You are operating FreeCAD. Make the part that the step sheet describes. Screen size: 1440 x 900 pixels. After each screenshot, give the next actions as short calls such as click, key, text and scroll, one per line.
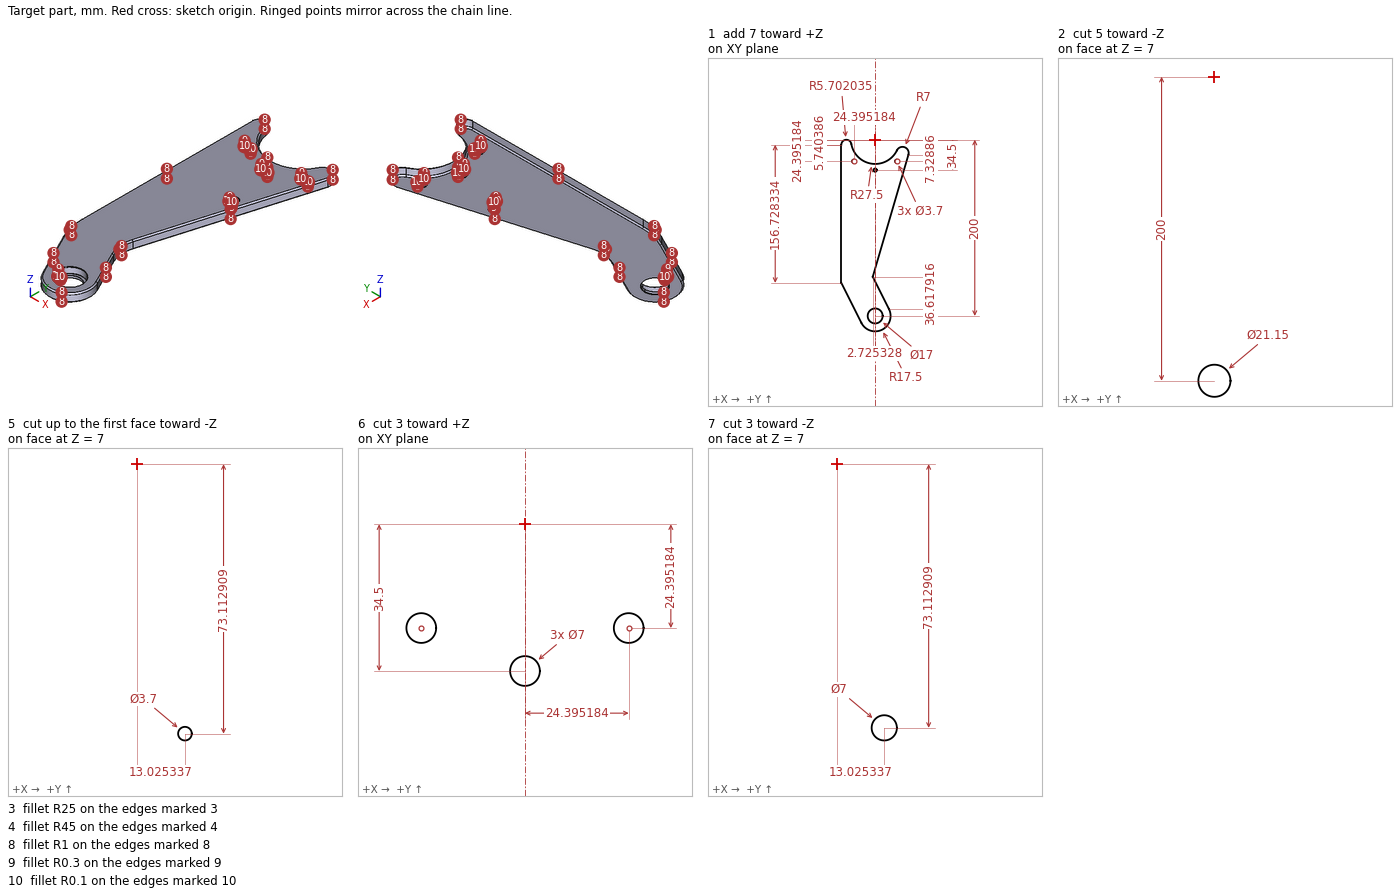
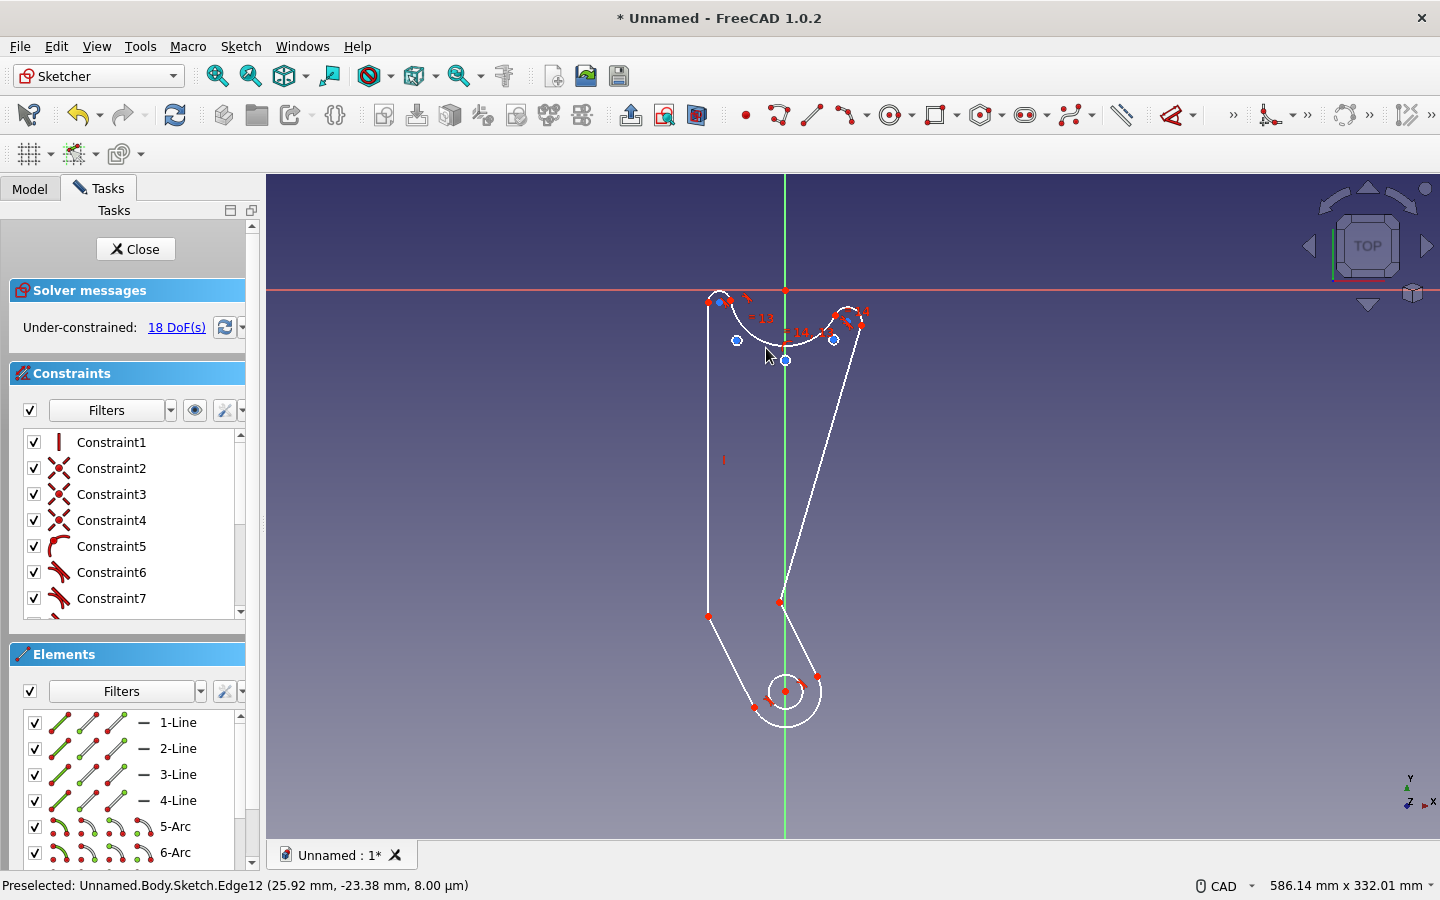
click(786, 692)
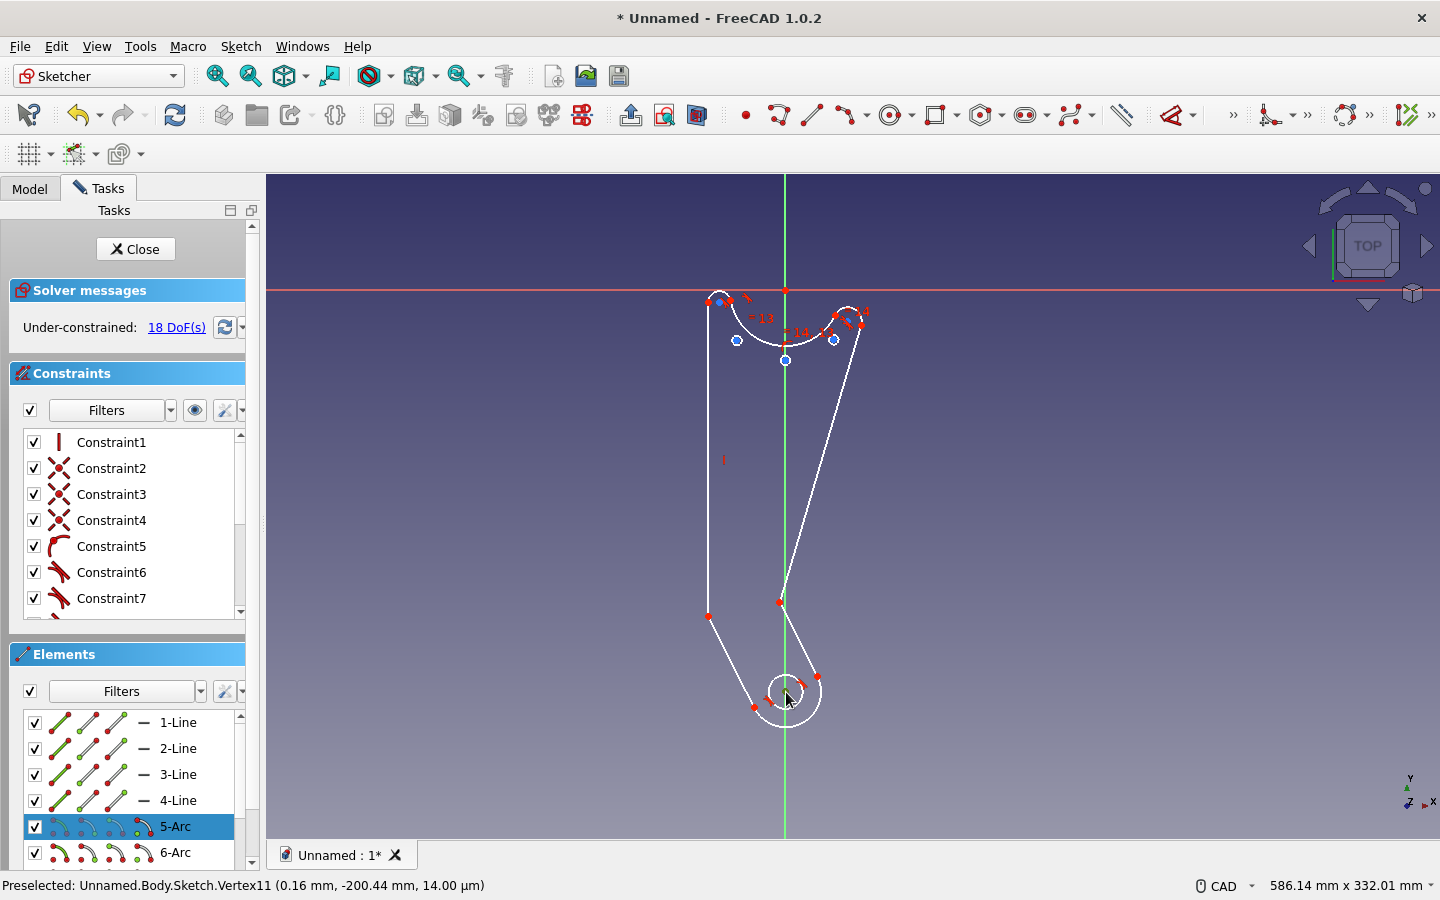
click(785, 768)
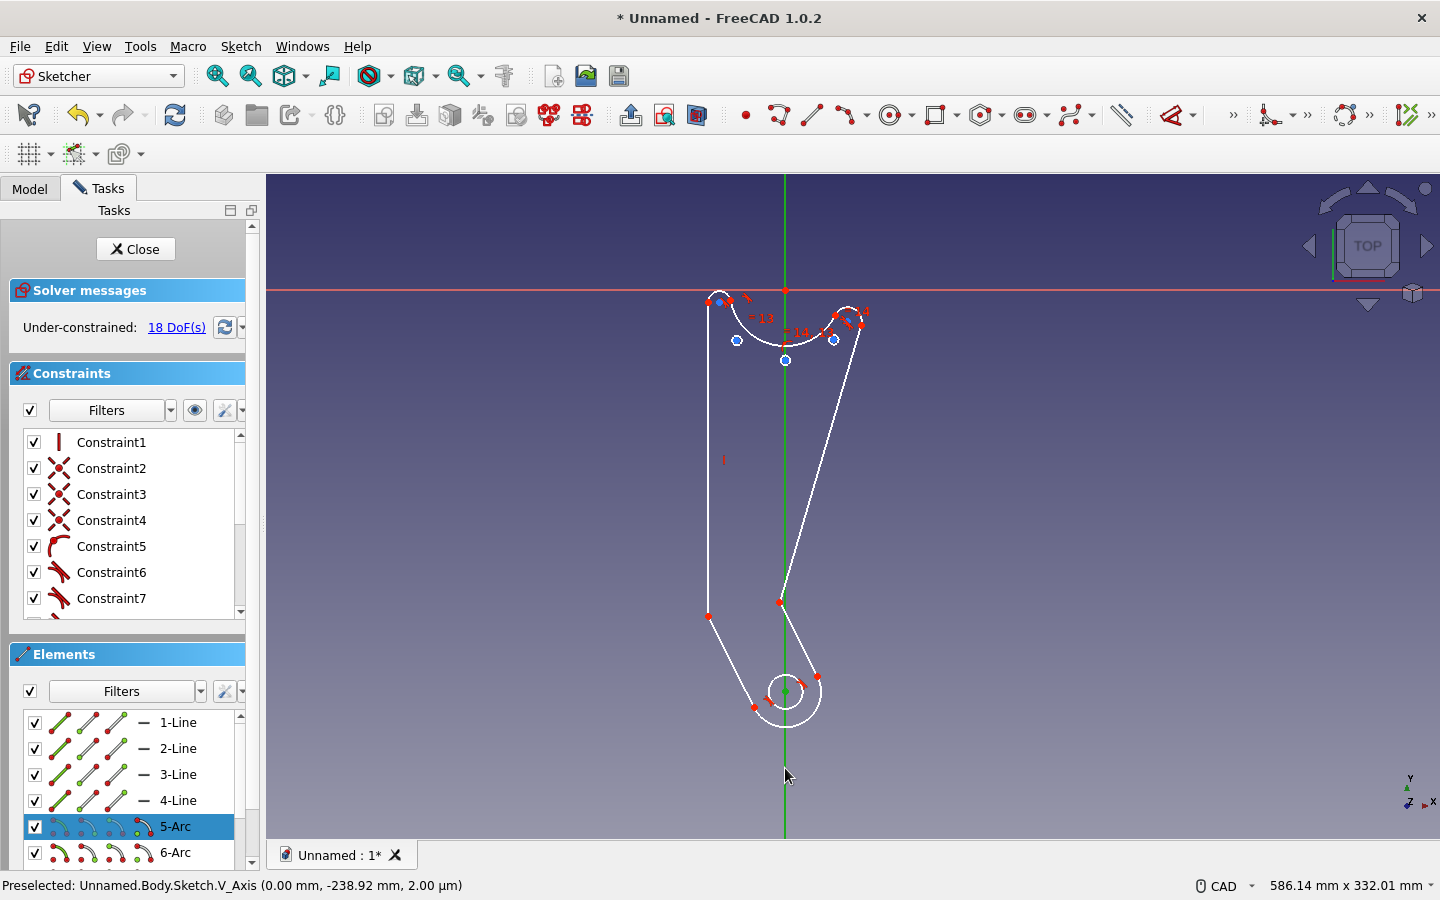
key(c)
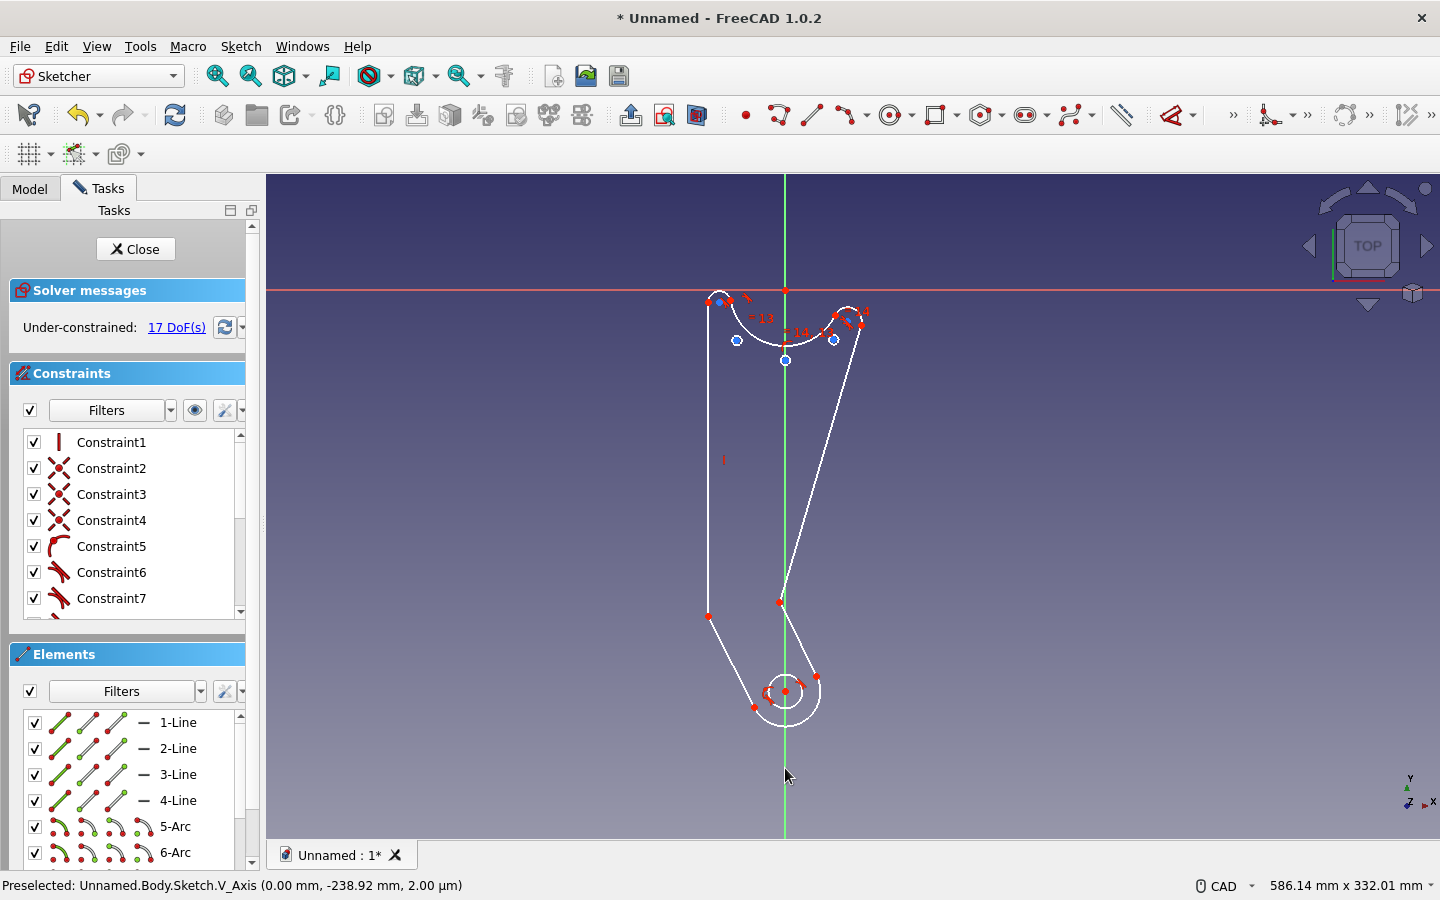
click(737, 341)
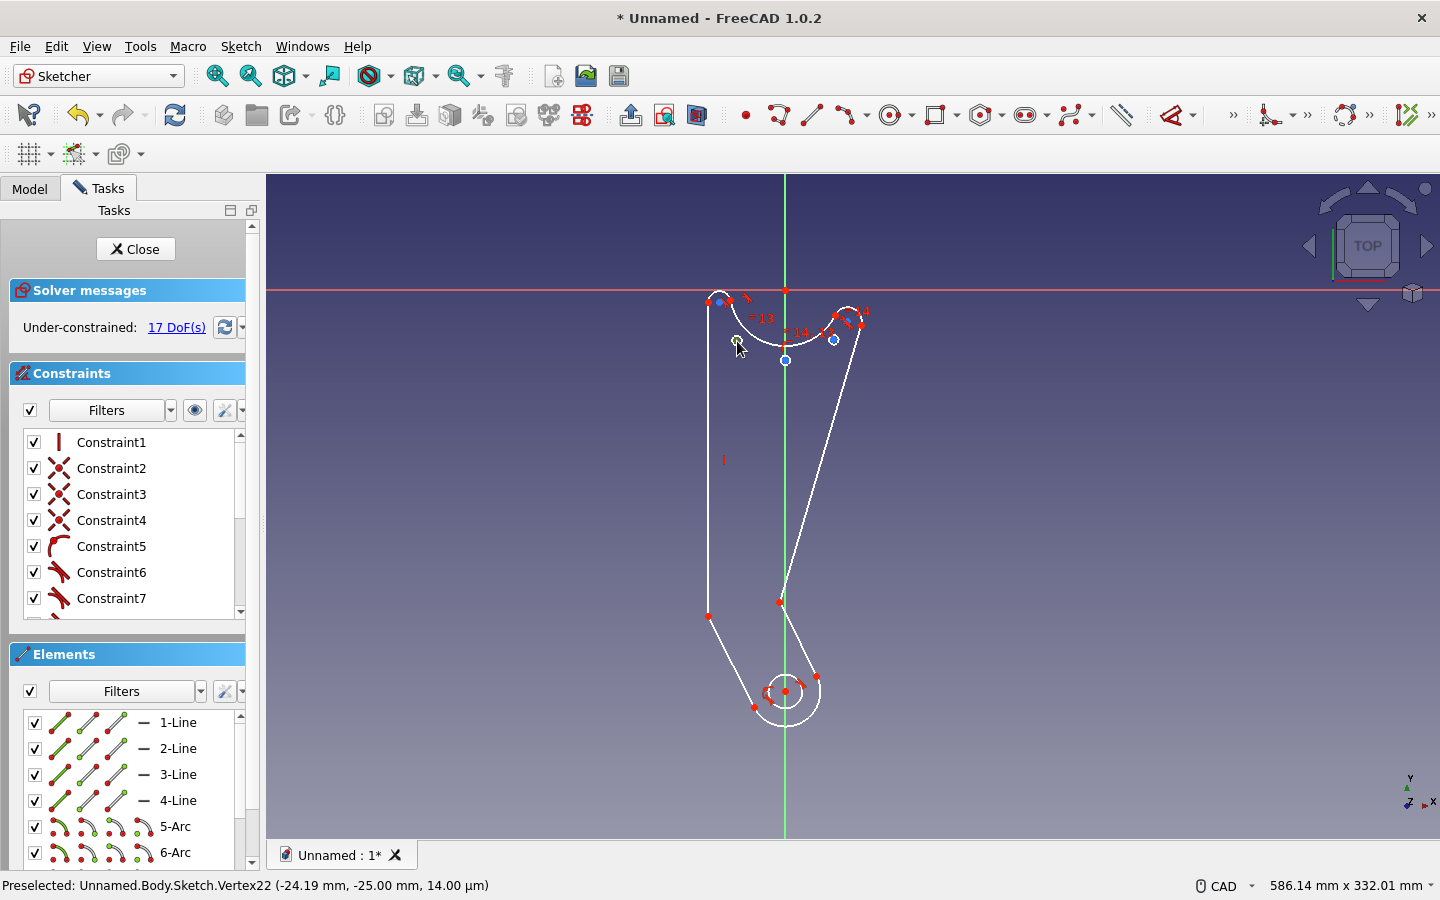
click(834, 340)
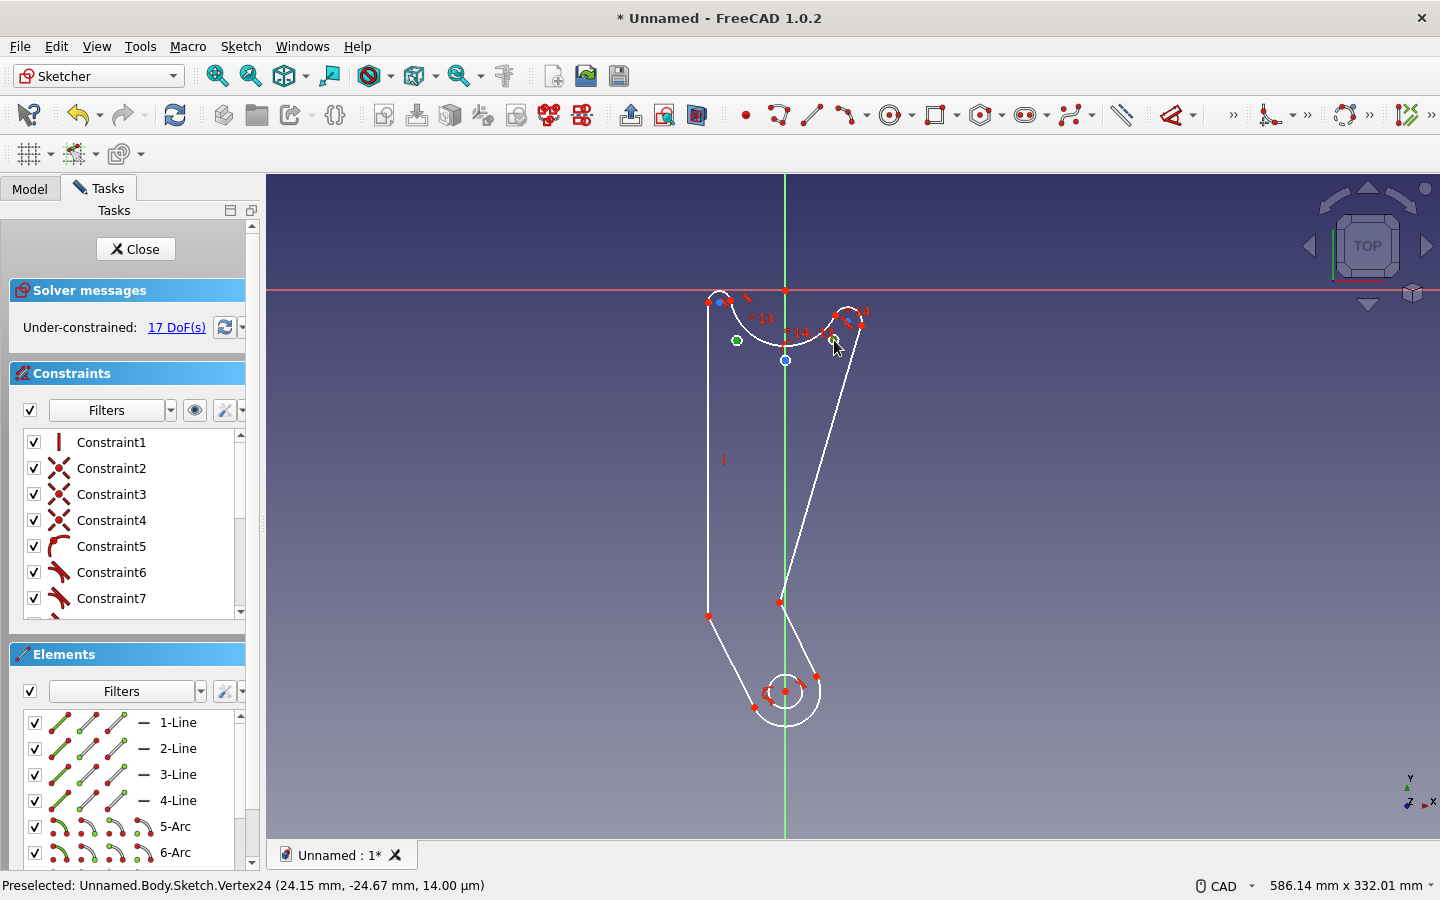
click(785, 768)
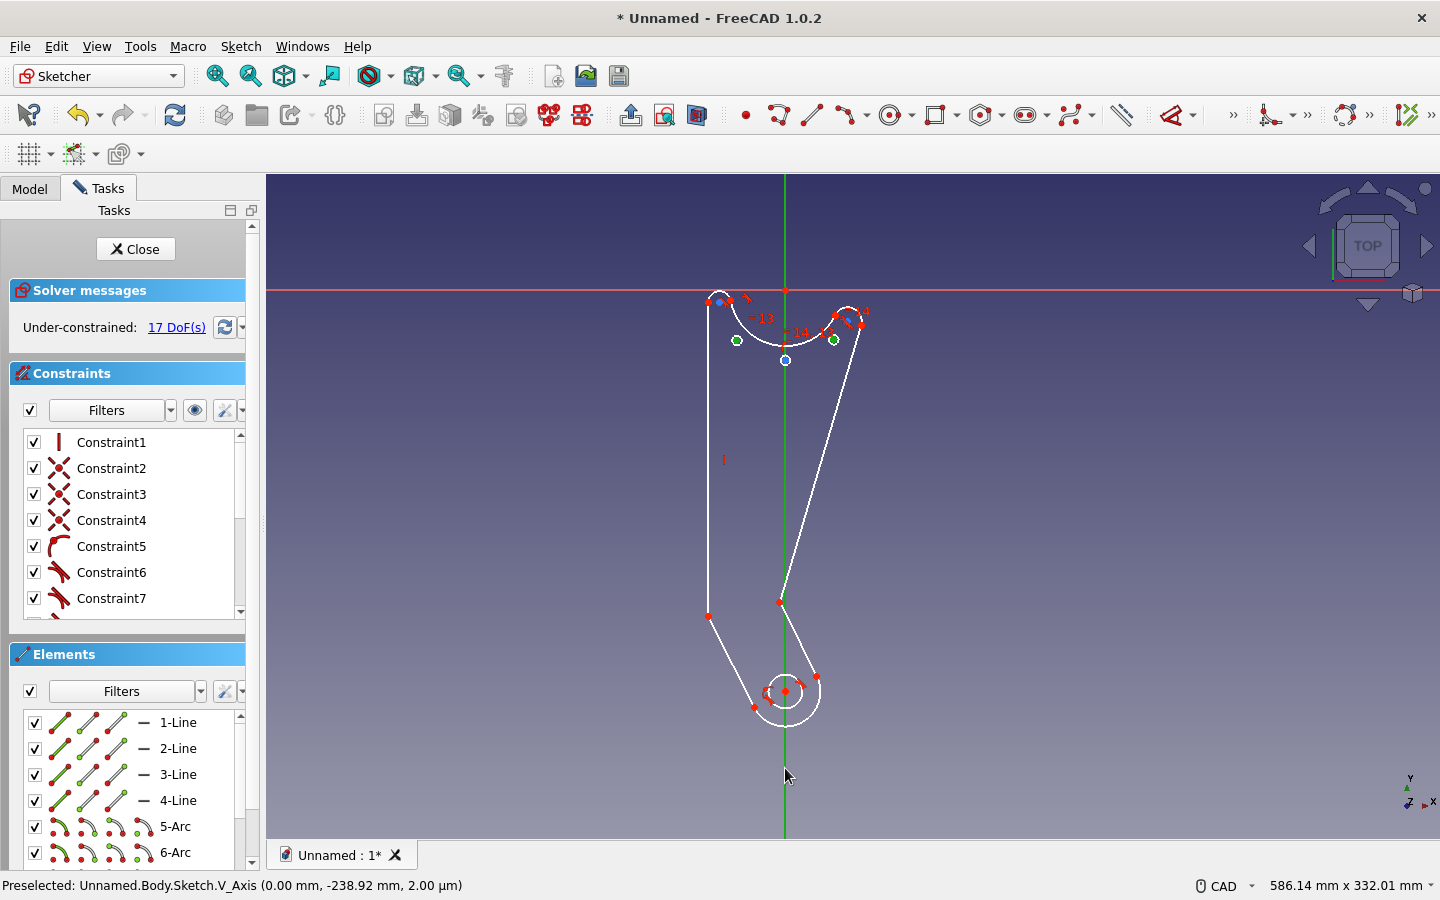
key(s)